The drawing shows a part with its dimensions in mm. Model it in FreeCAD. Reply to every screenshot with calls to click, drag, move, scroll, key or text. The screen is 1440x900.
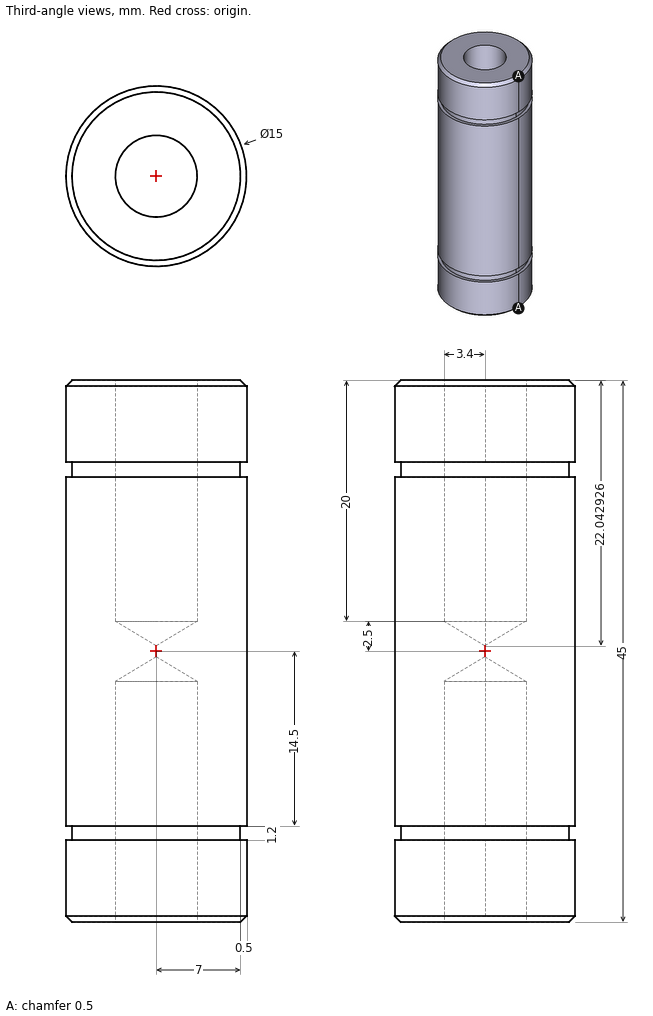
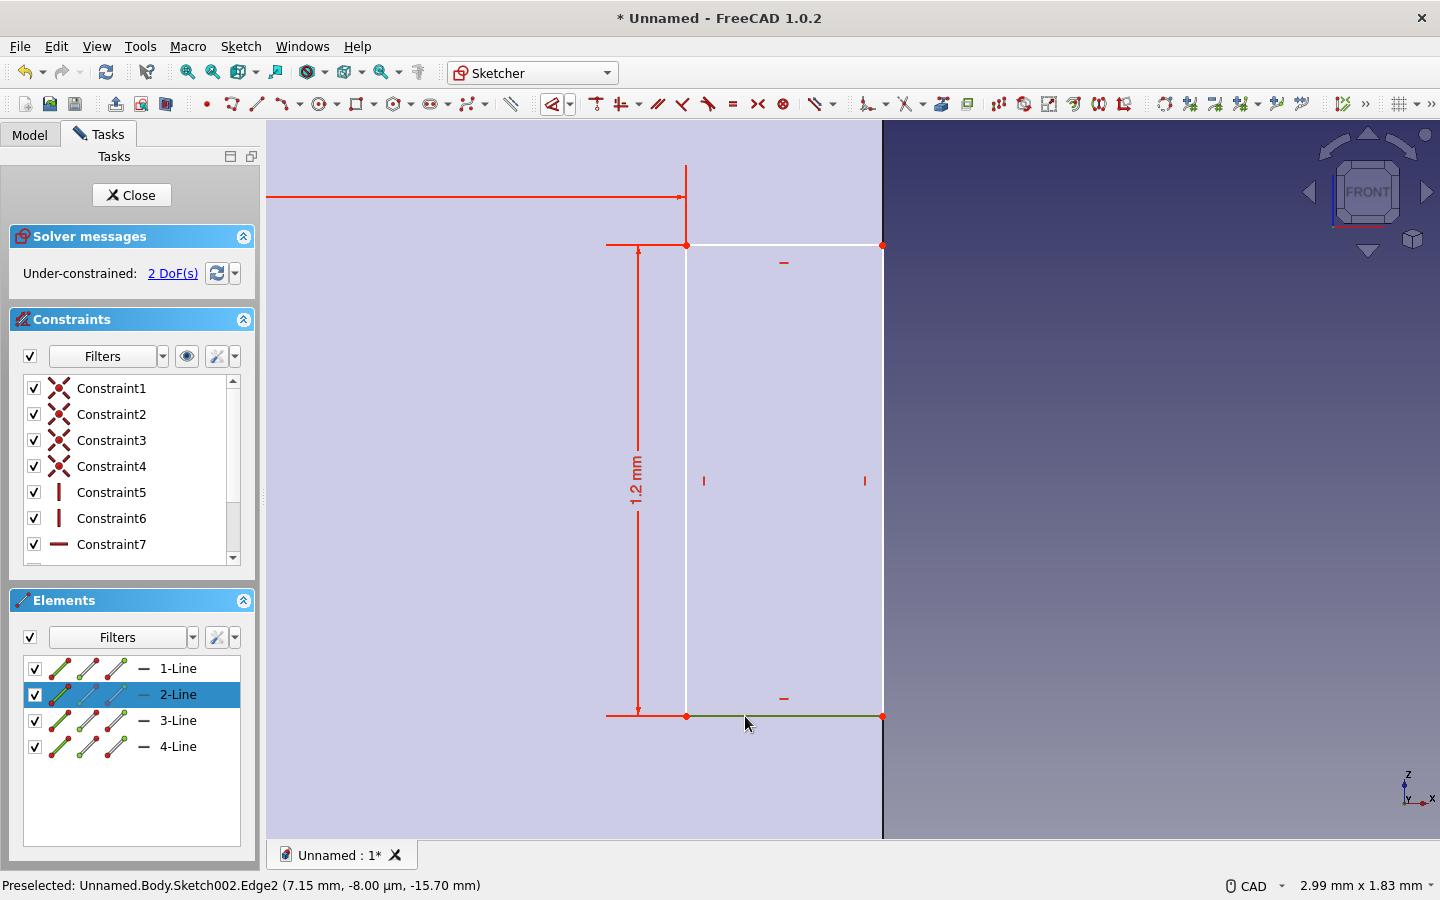
key(l)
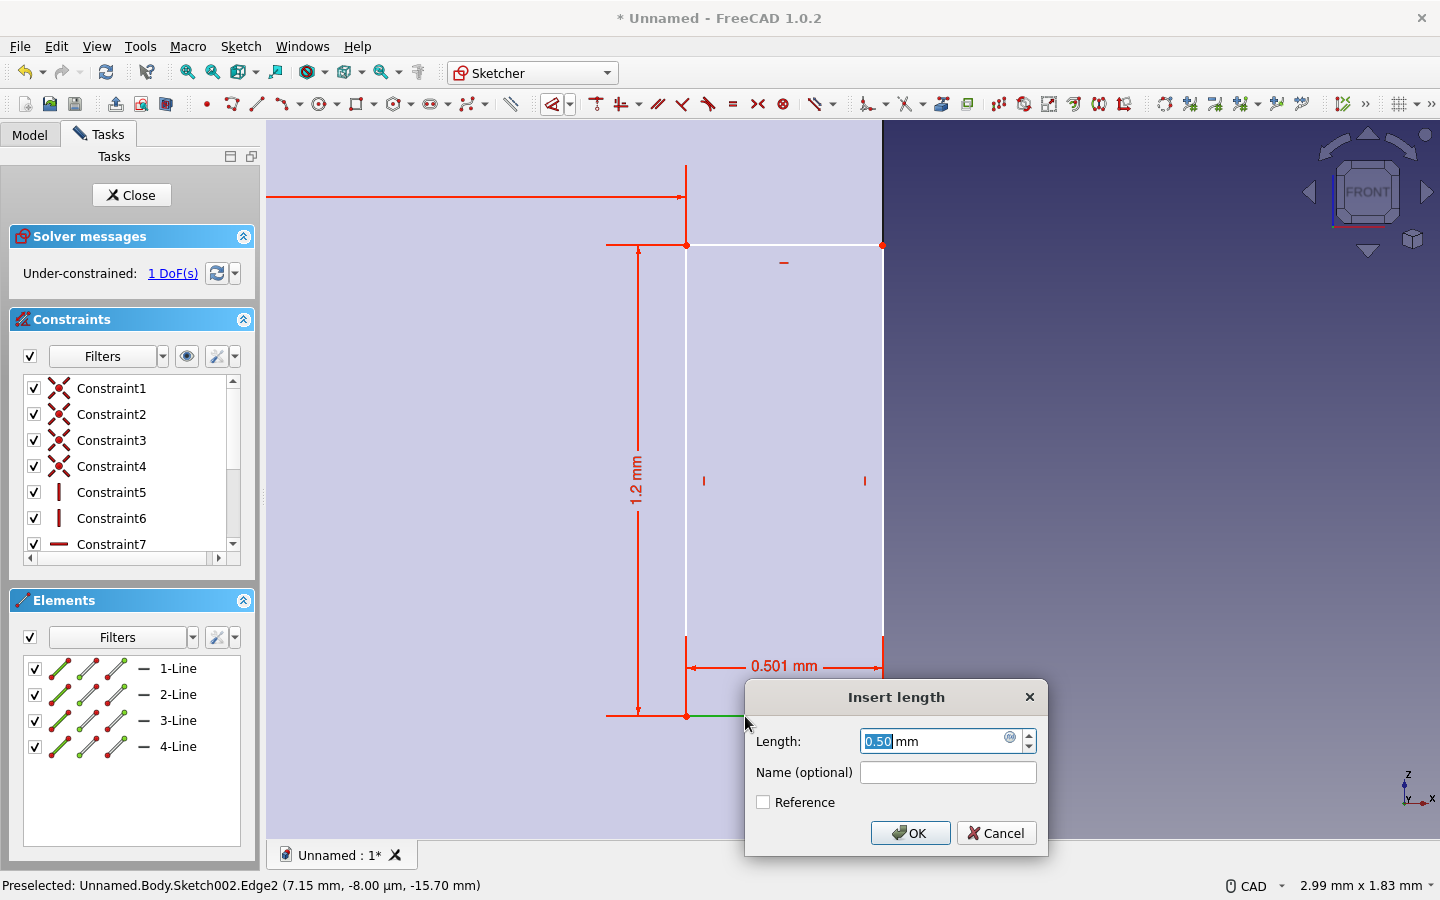
text(0.5)
key(Return)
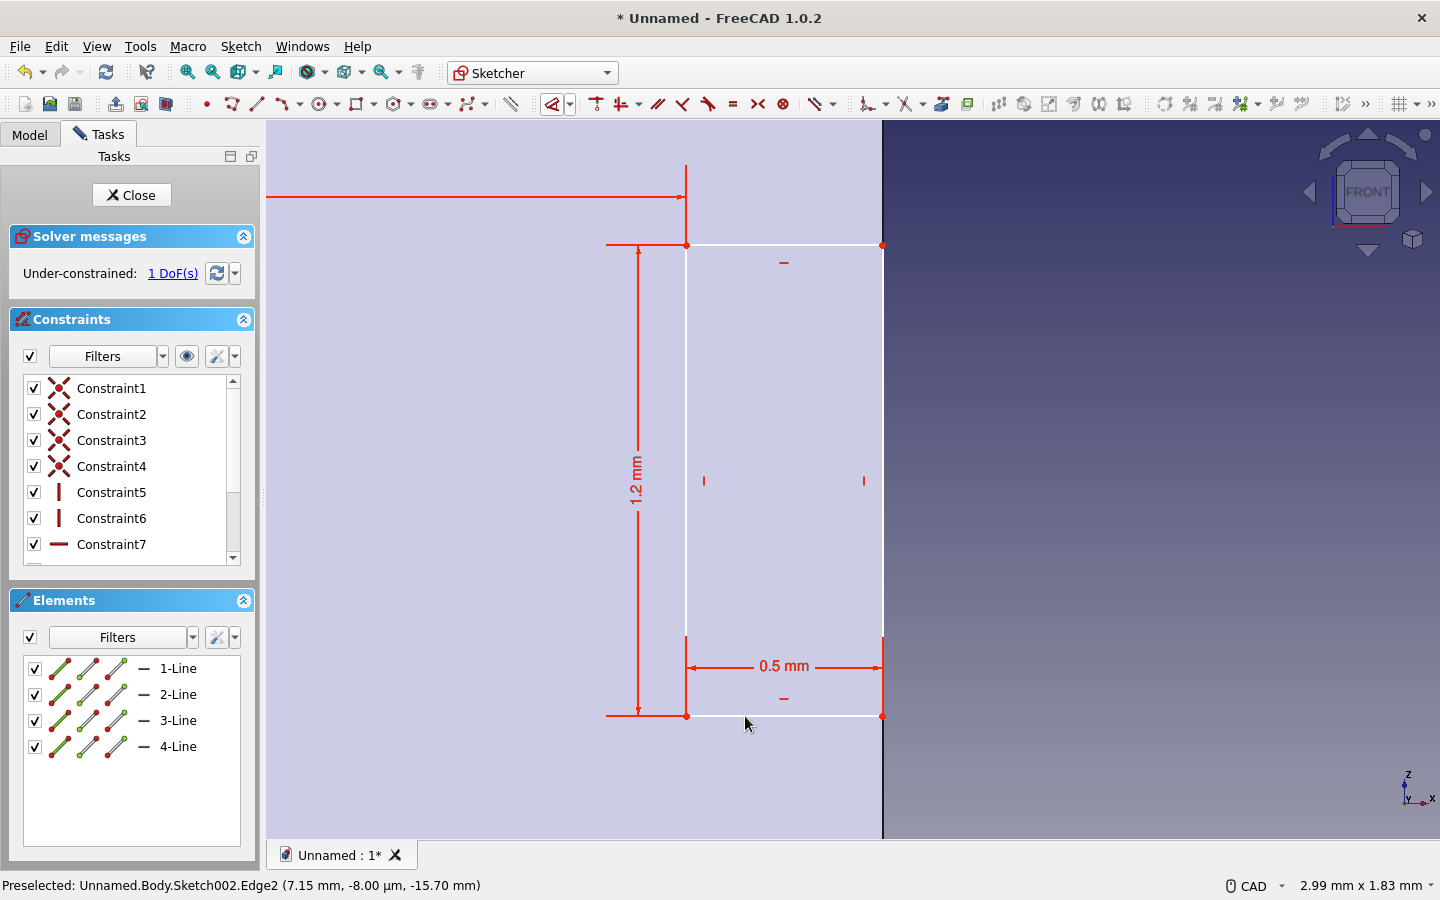
click(686, 245)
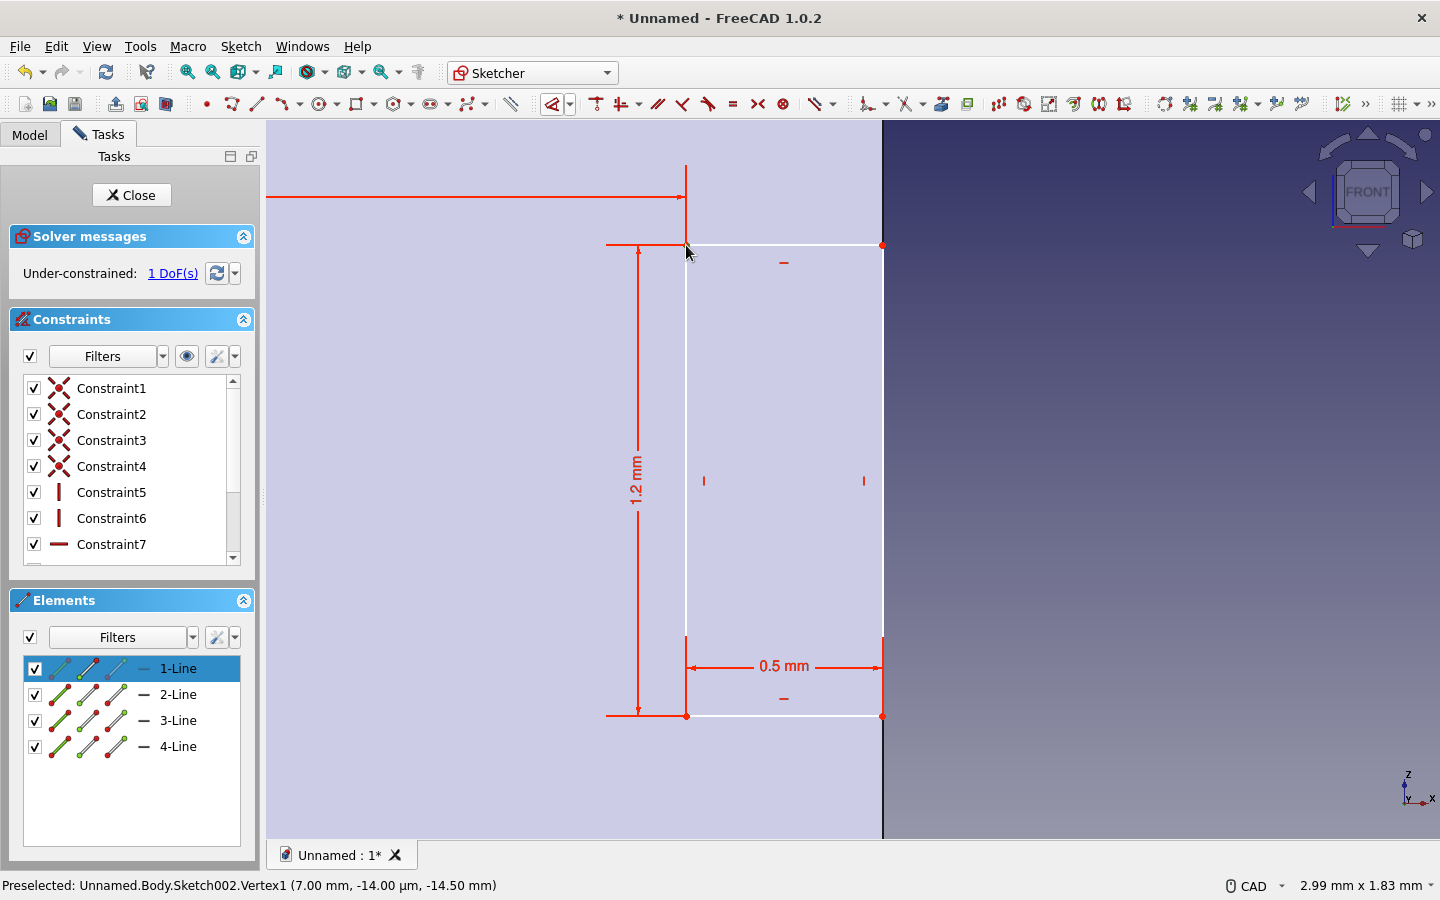
key(i)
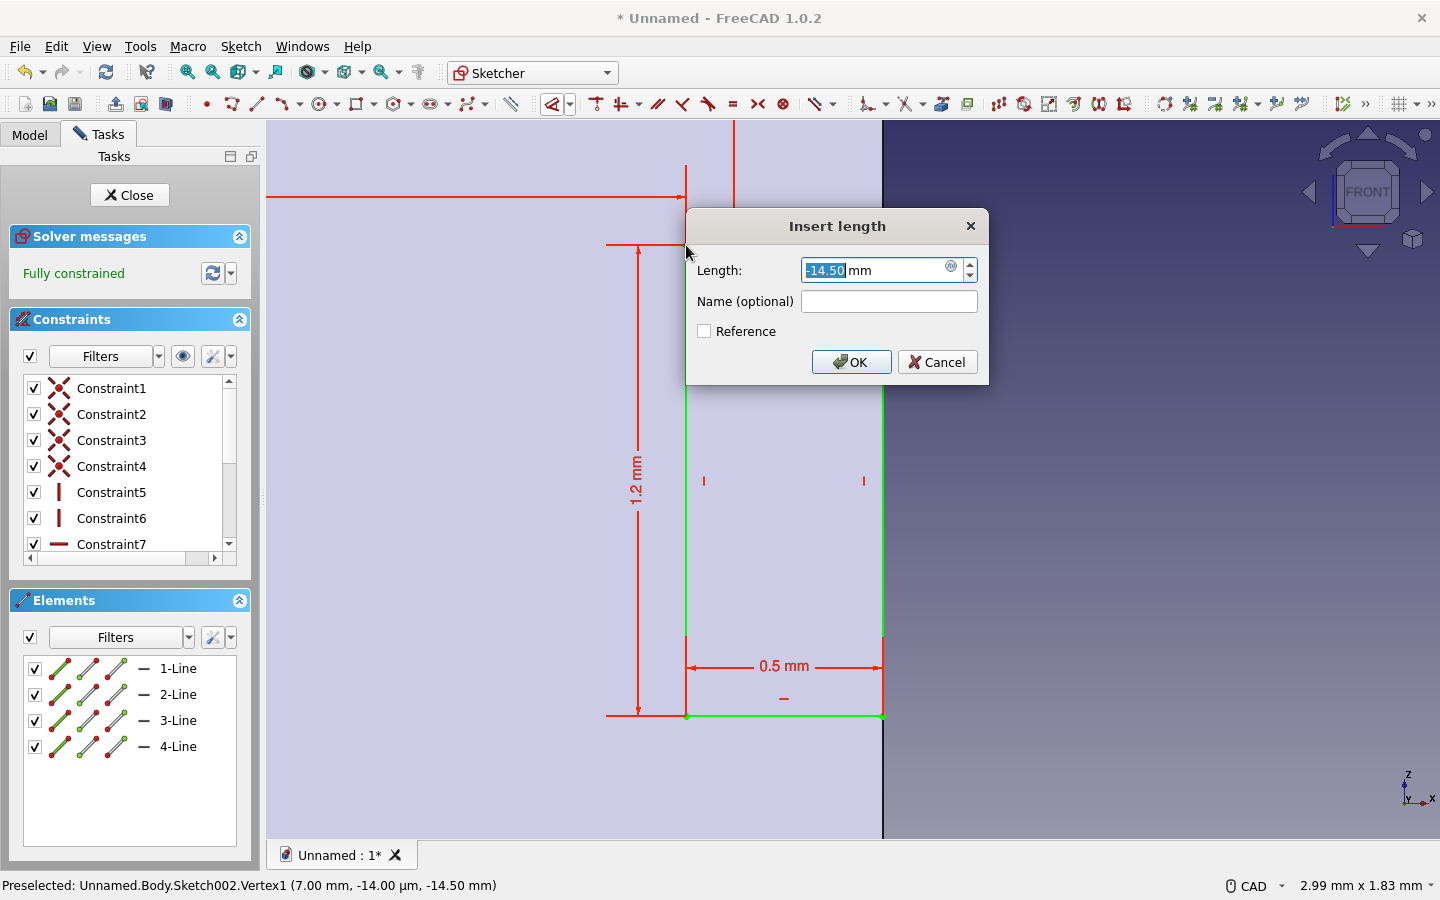
text(-14.5)
key(Return)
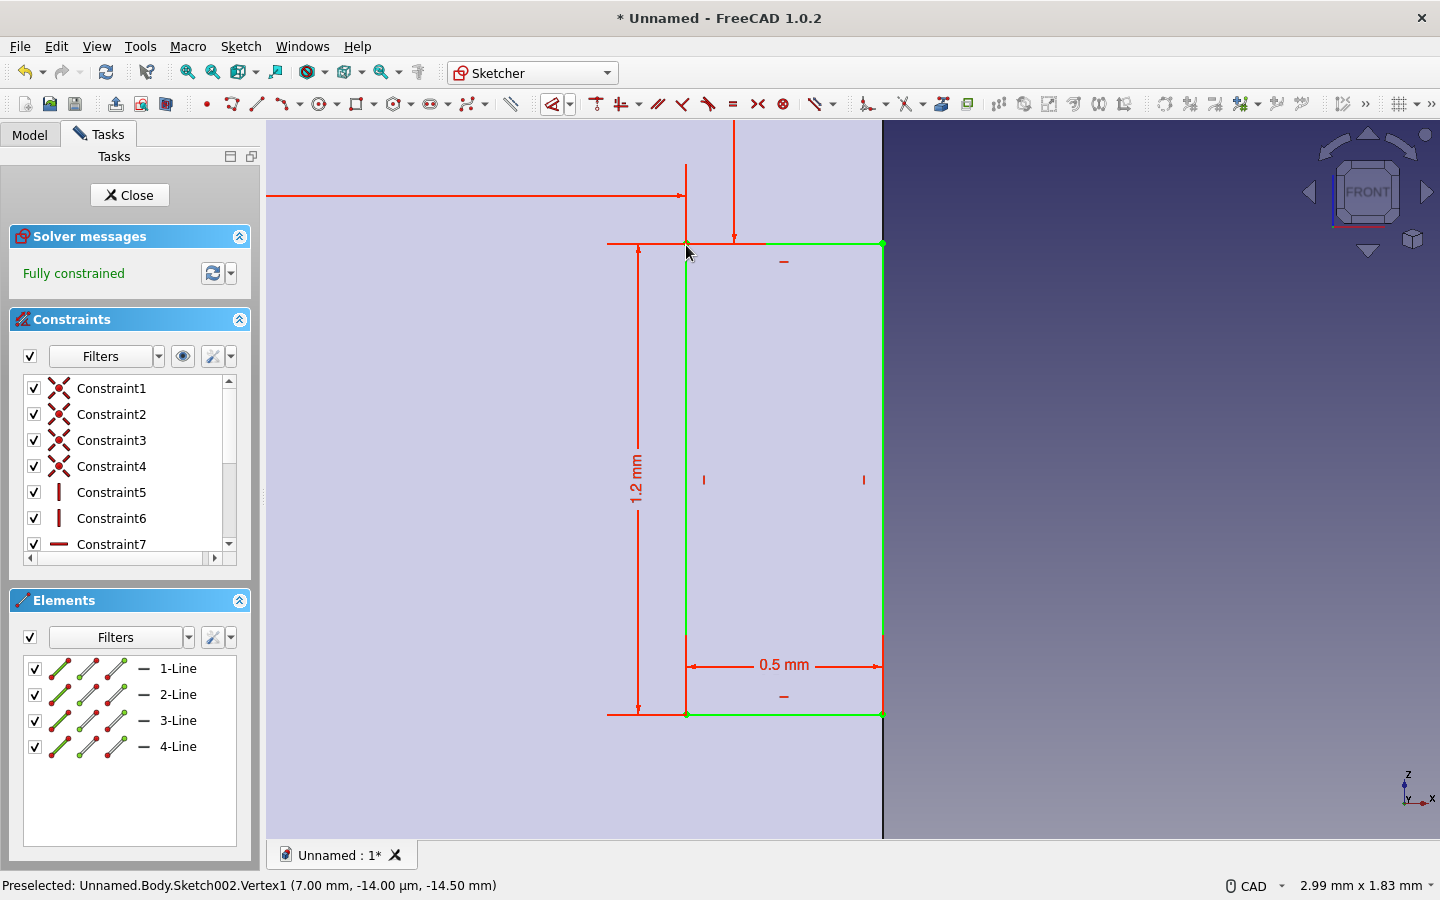
click(130, 195)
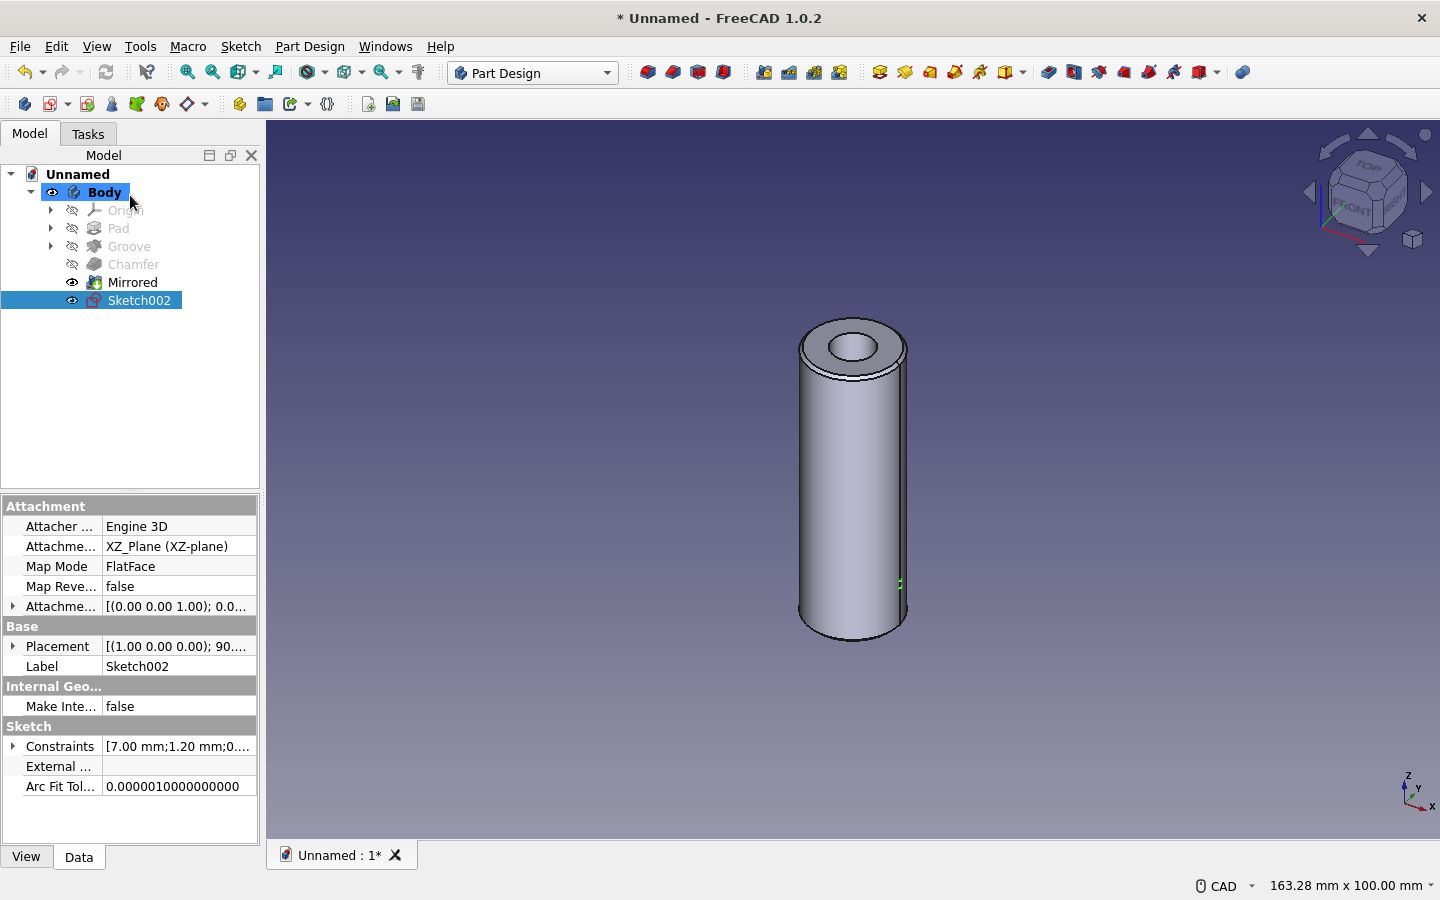
click(1099, 72)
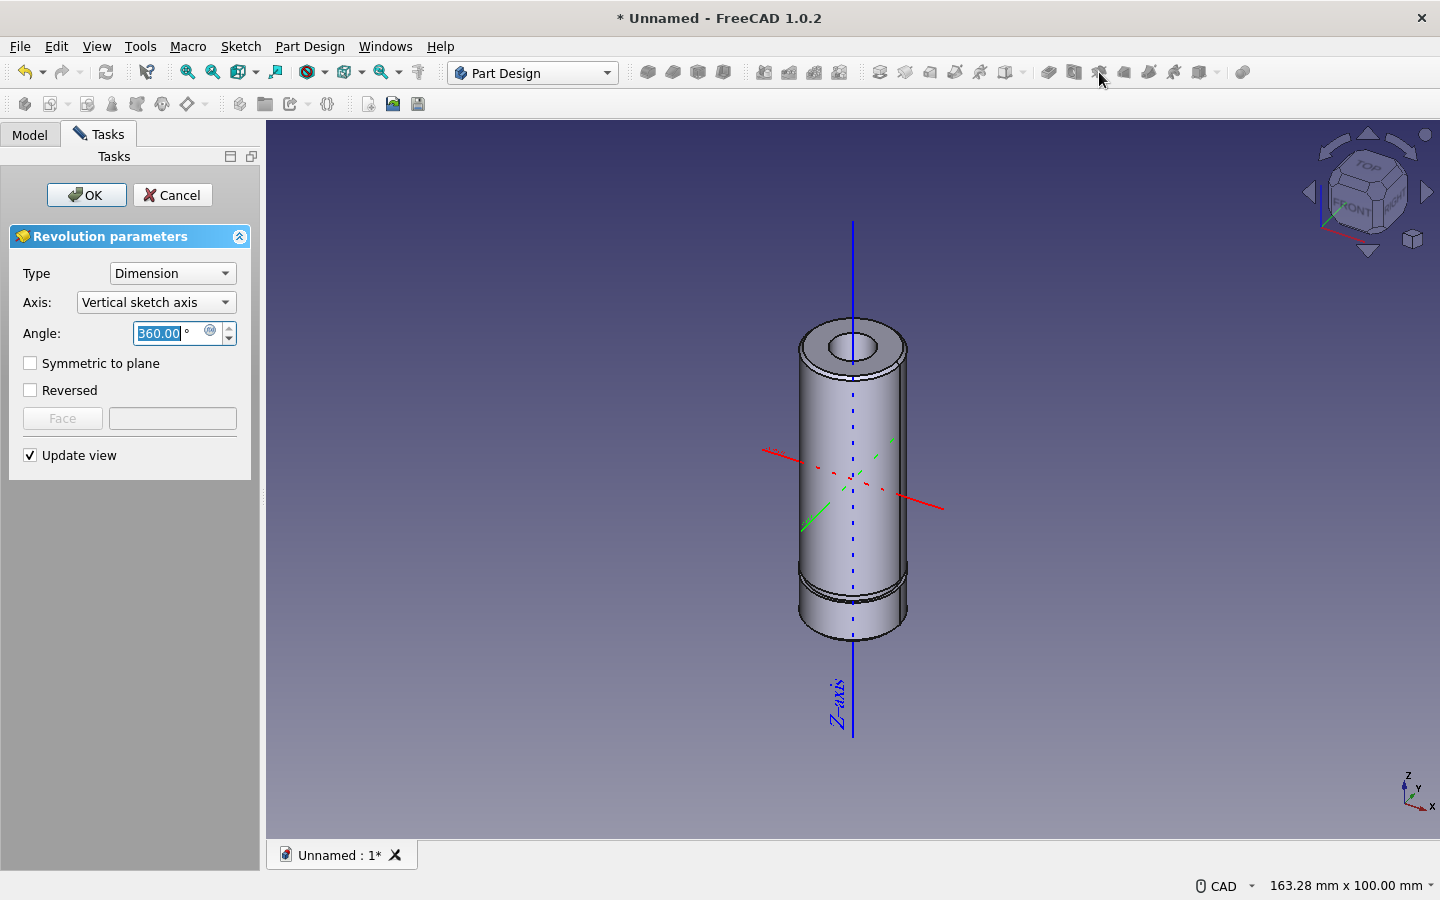
click(87, 195)